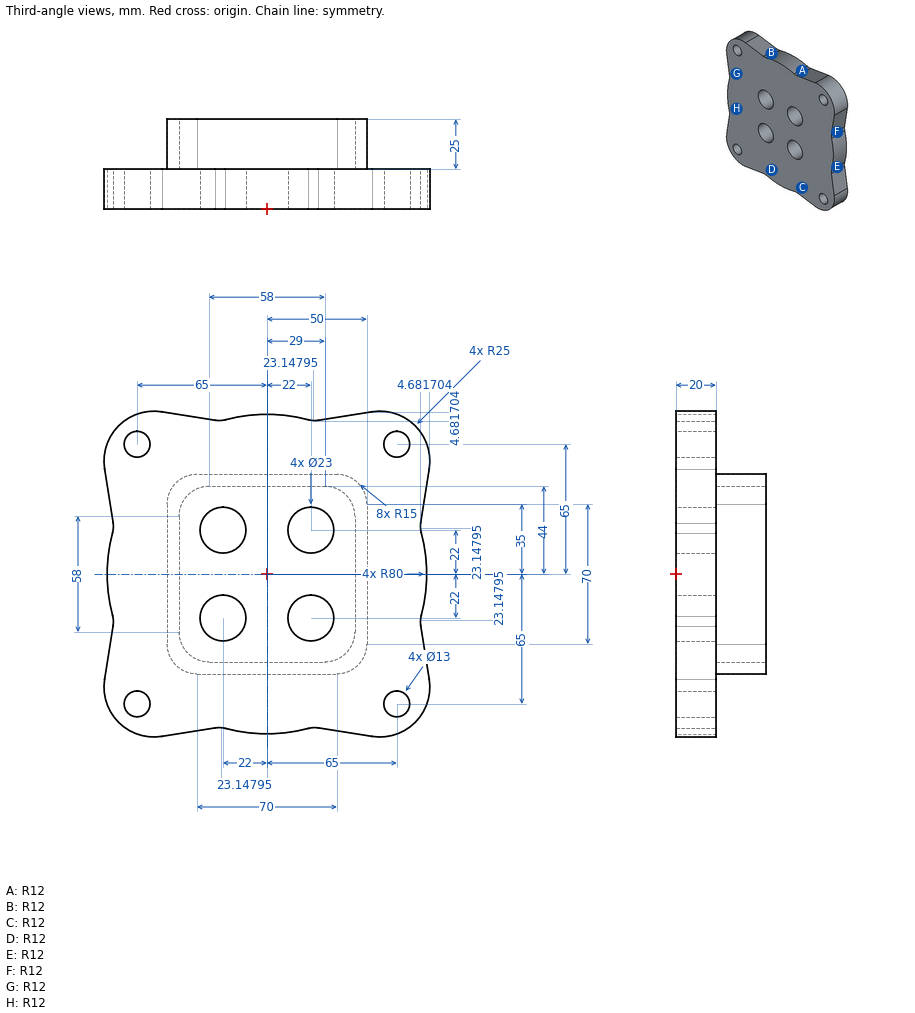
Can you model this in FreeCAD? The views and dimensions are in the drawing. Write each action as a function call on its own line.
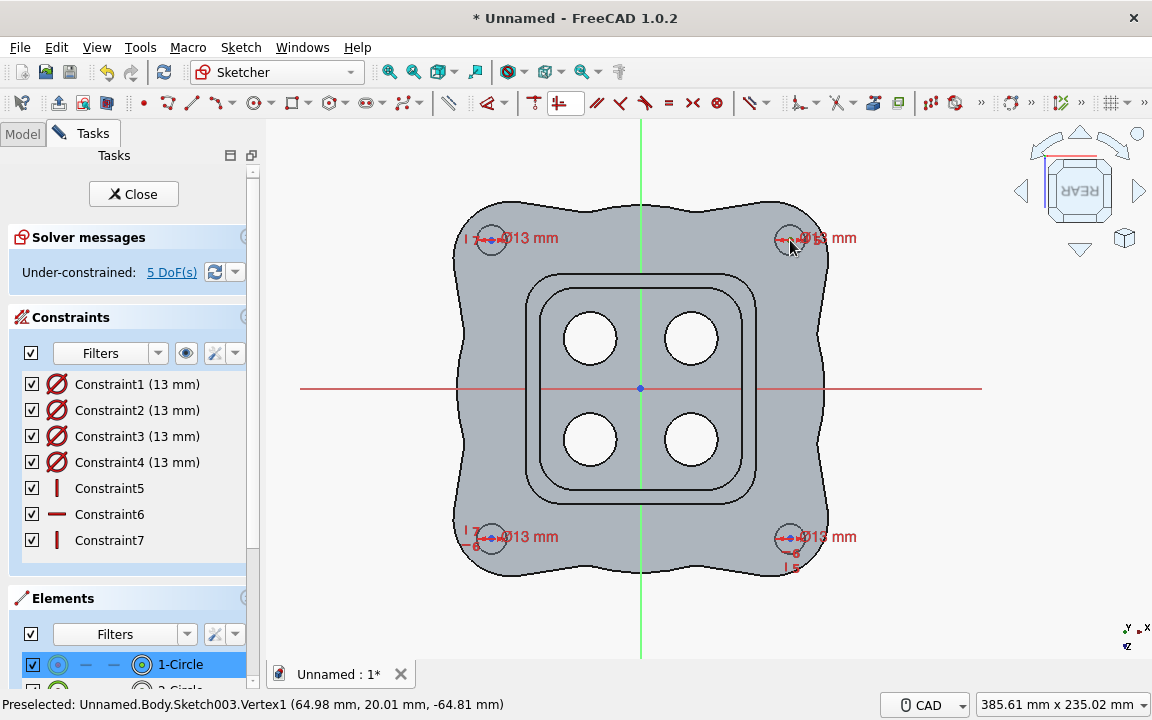
click(492, 240)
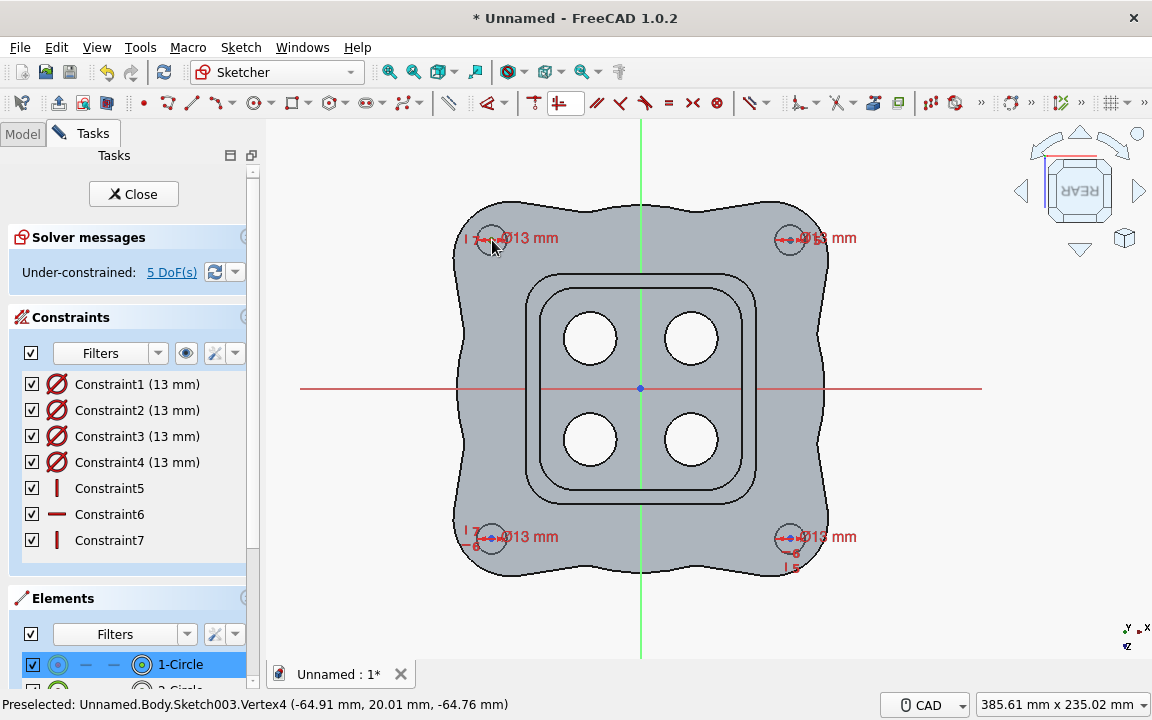
click(578, 104)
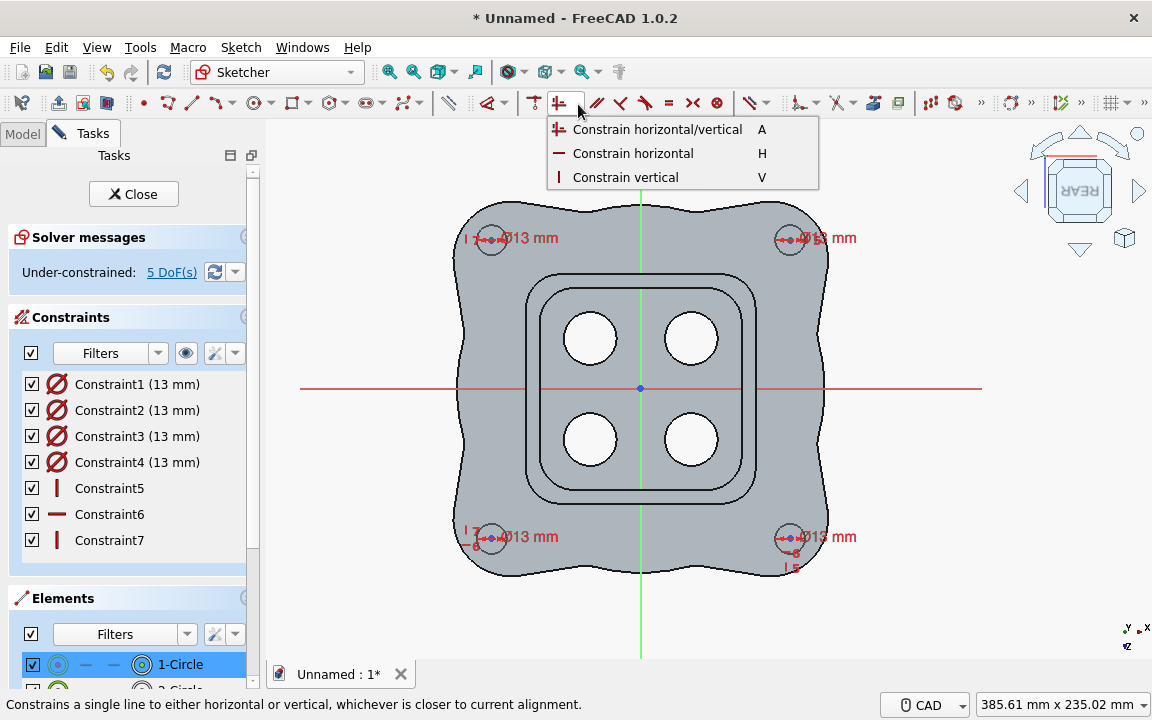
click(683, 153)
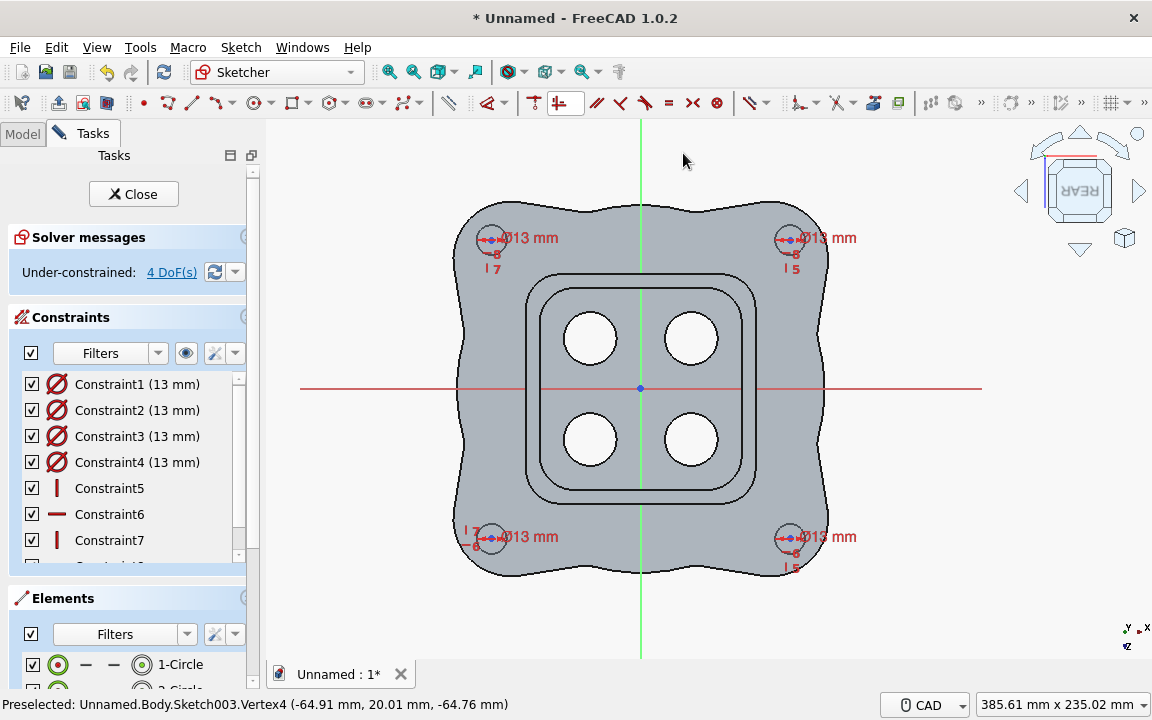
click(488, 104)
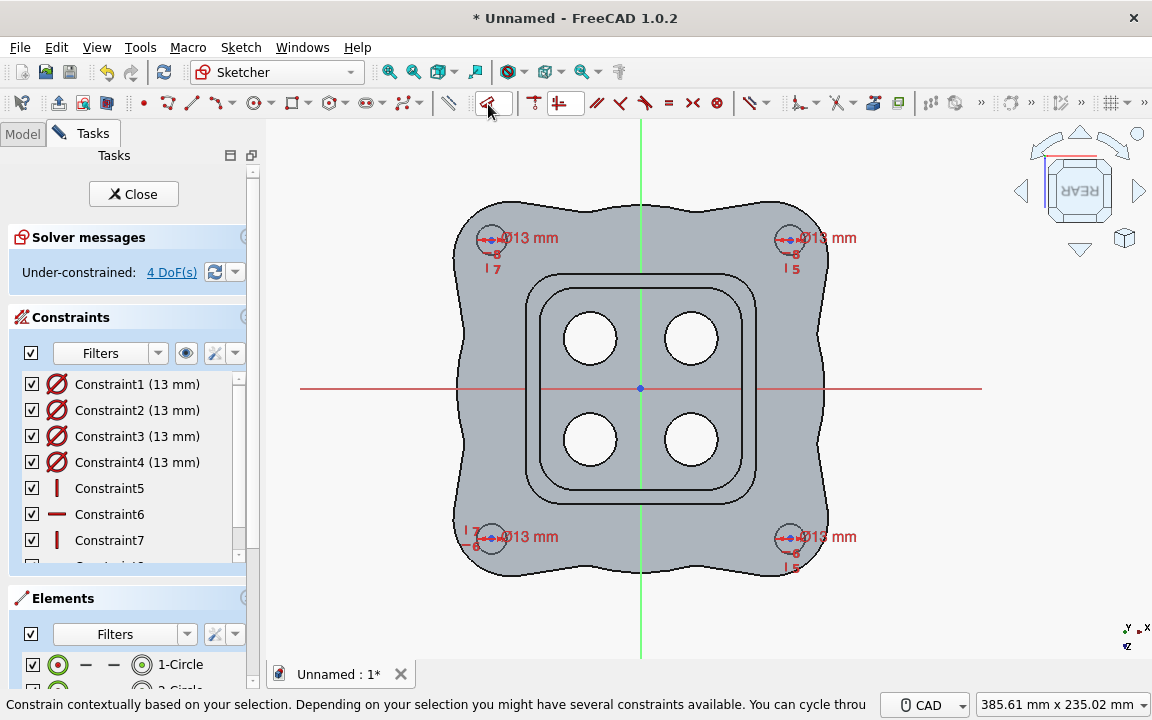
click(790, 240)
click(715, 206)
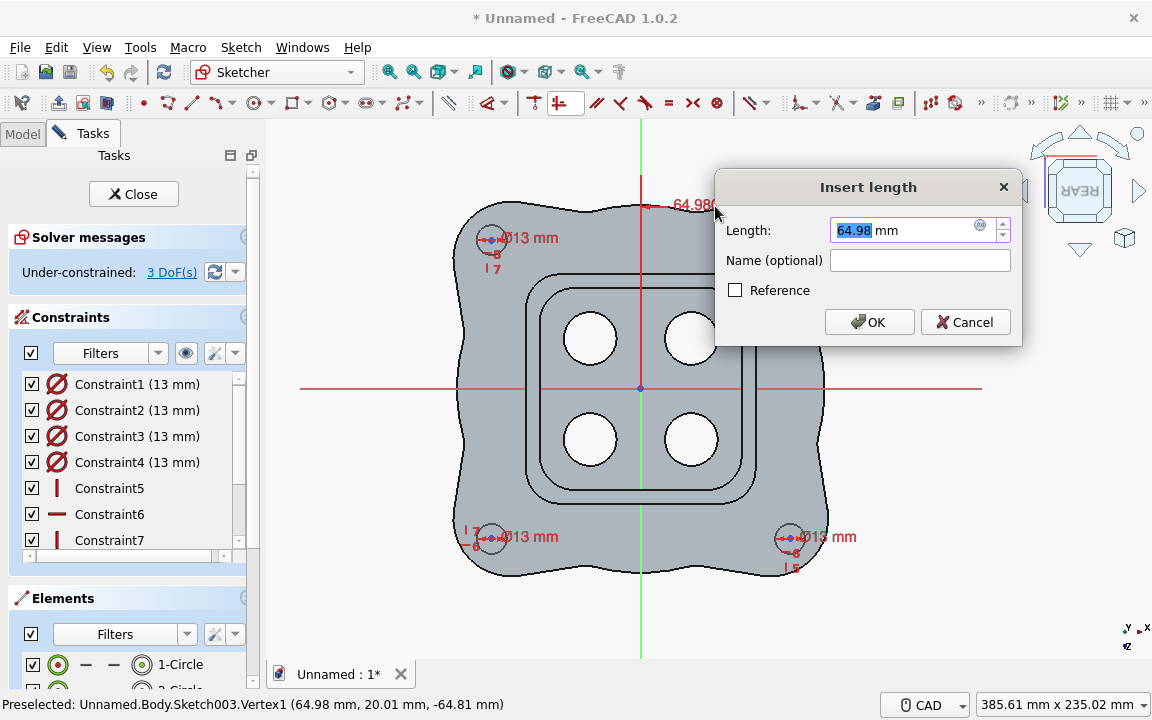
text(65)
key(Return)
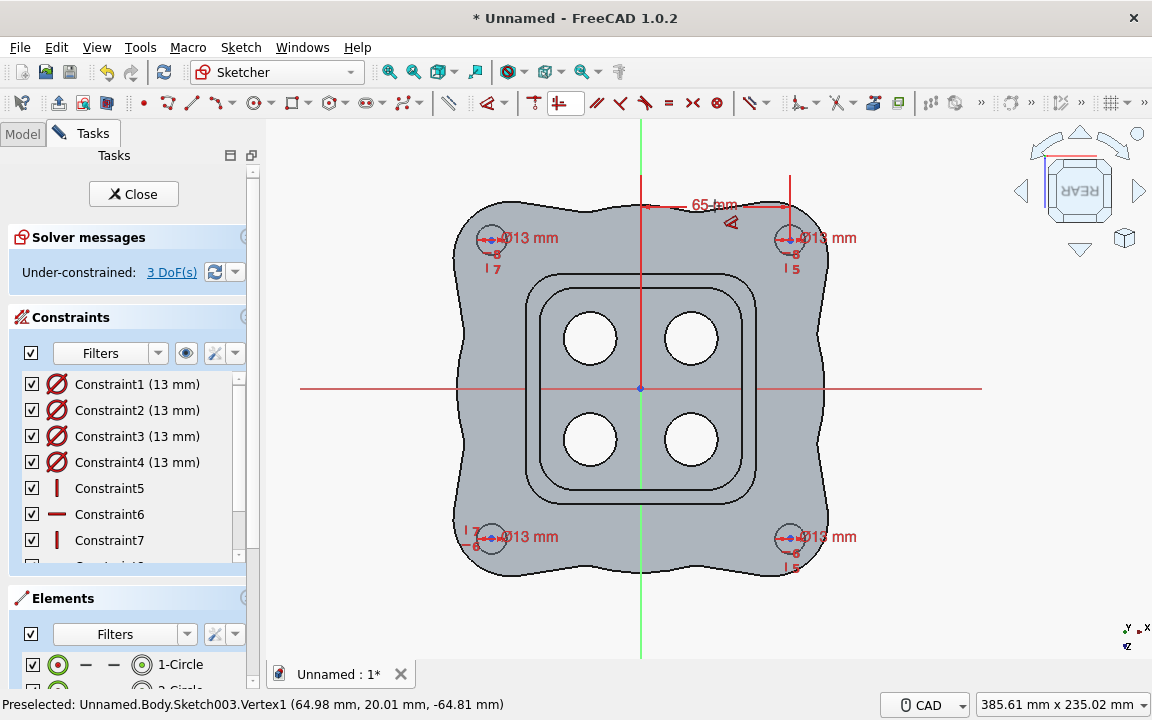
click(790, 240)
click(824, 315)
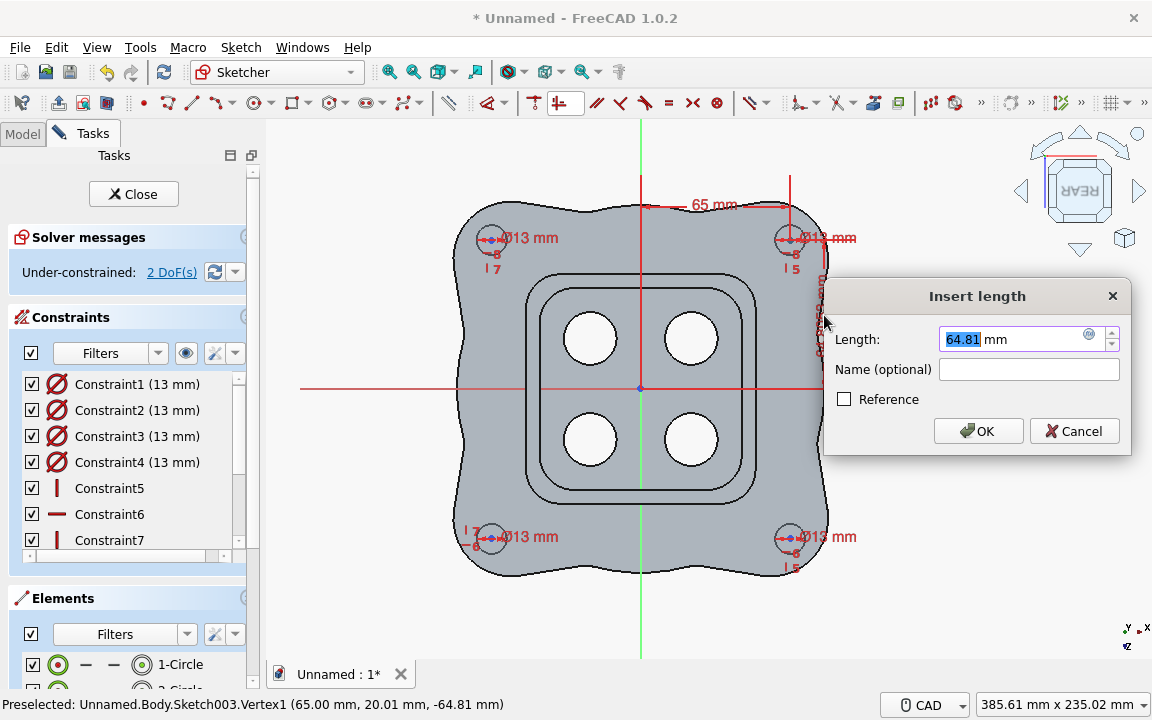
text(65)
key(Return)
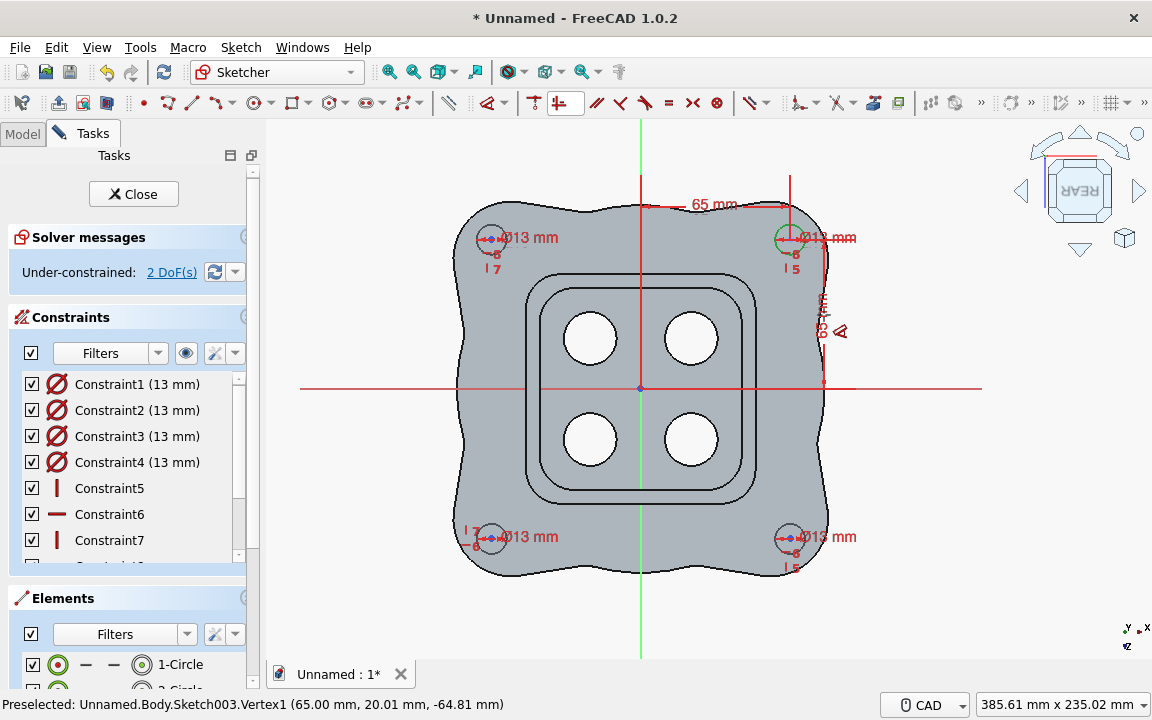
click(790, 539)
click(824, 464)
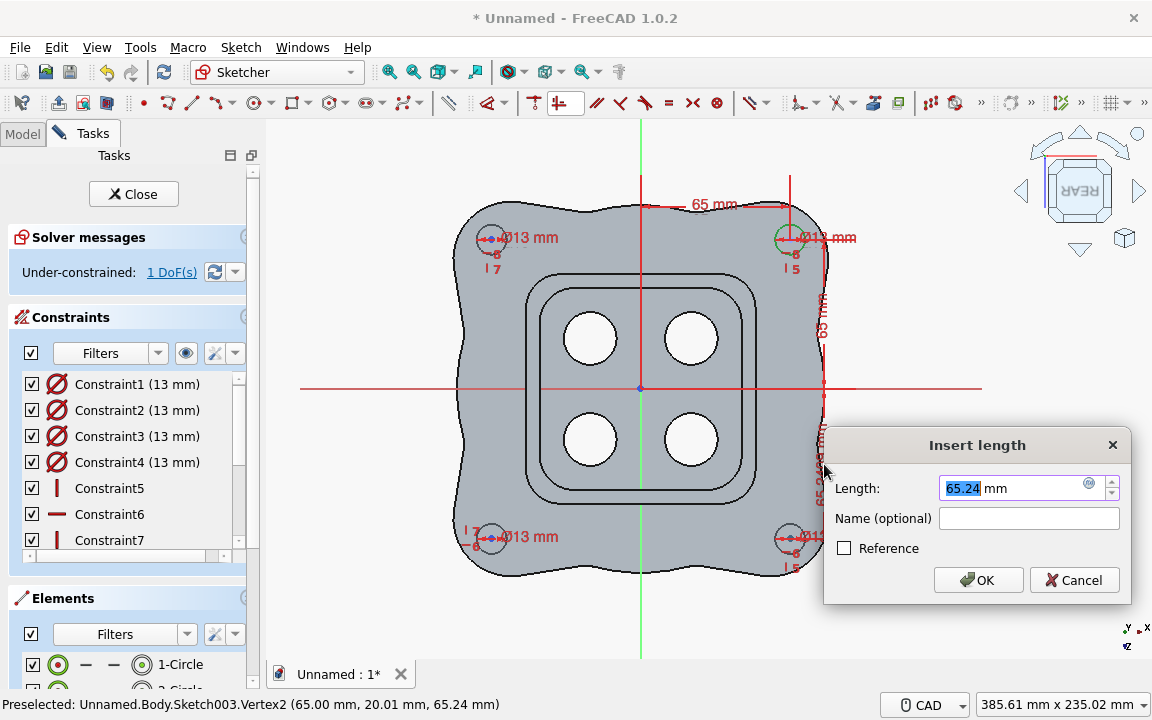
text(65)
key(Return)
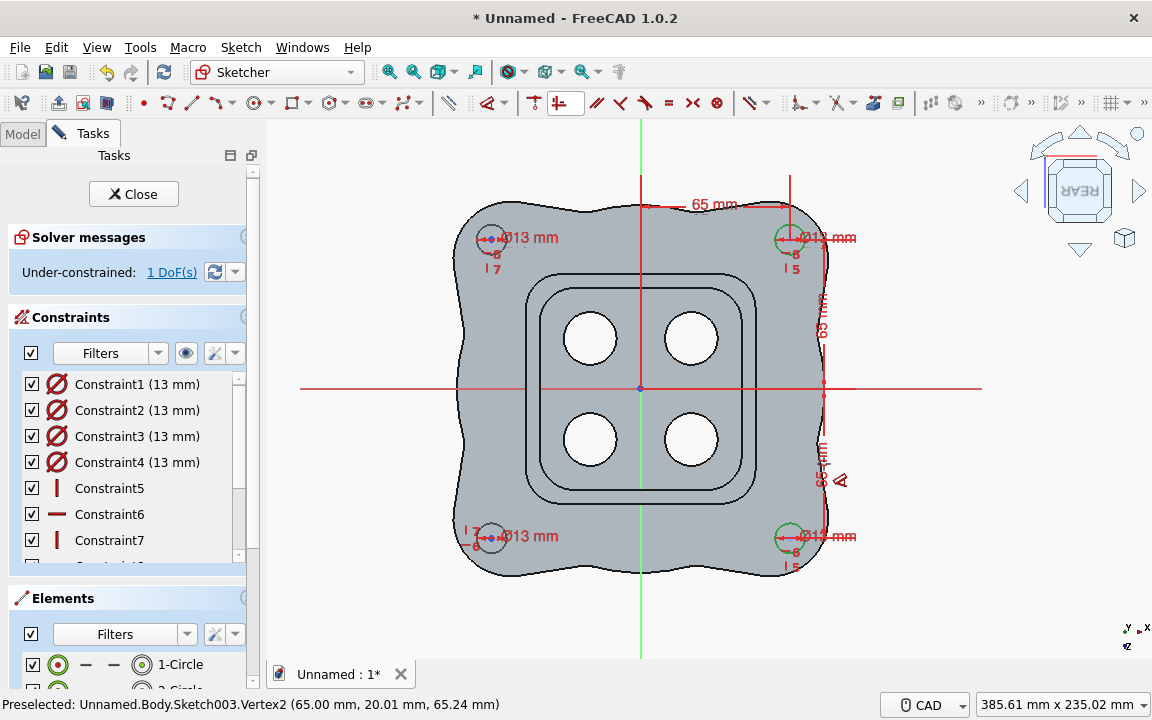
click(492, 538)
click(566, 572)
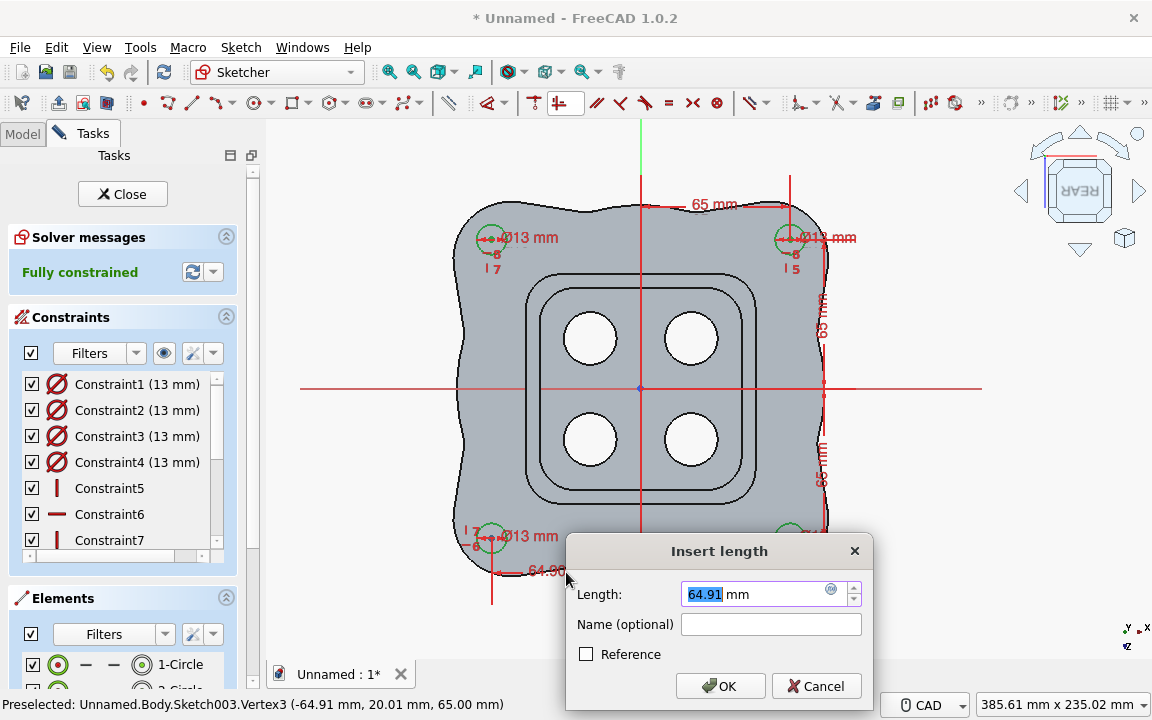
text(65)
key(Return)
key(Escape)